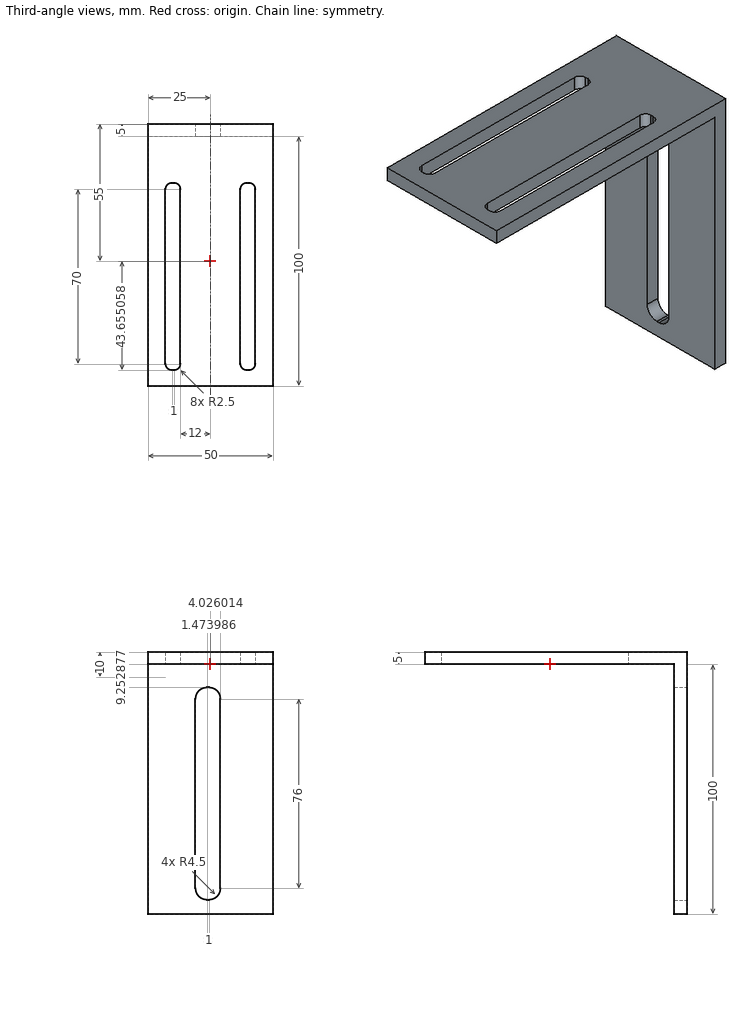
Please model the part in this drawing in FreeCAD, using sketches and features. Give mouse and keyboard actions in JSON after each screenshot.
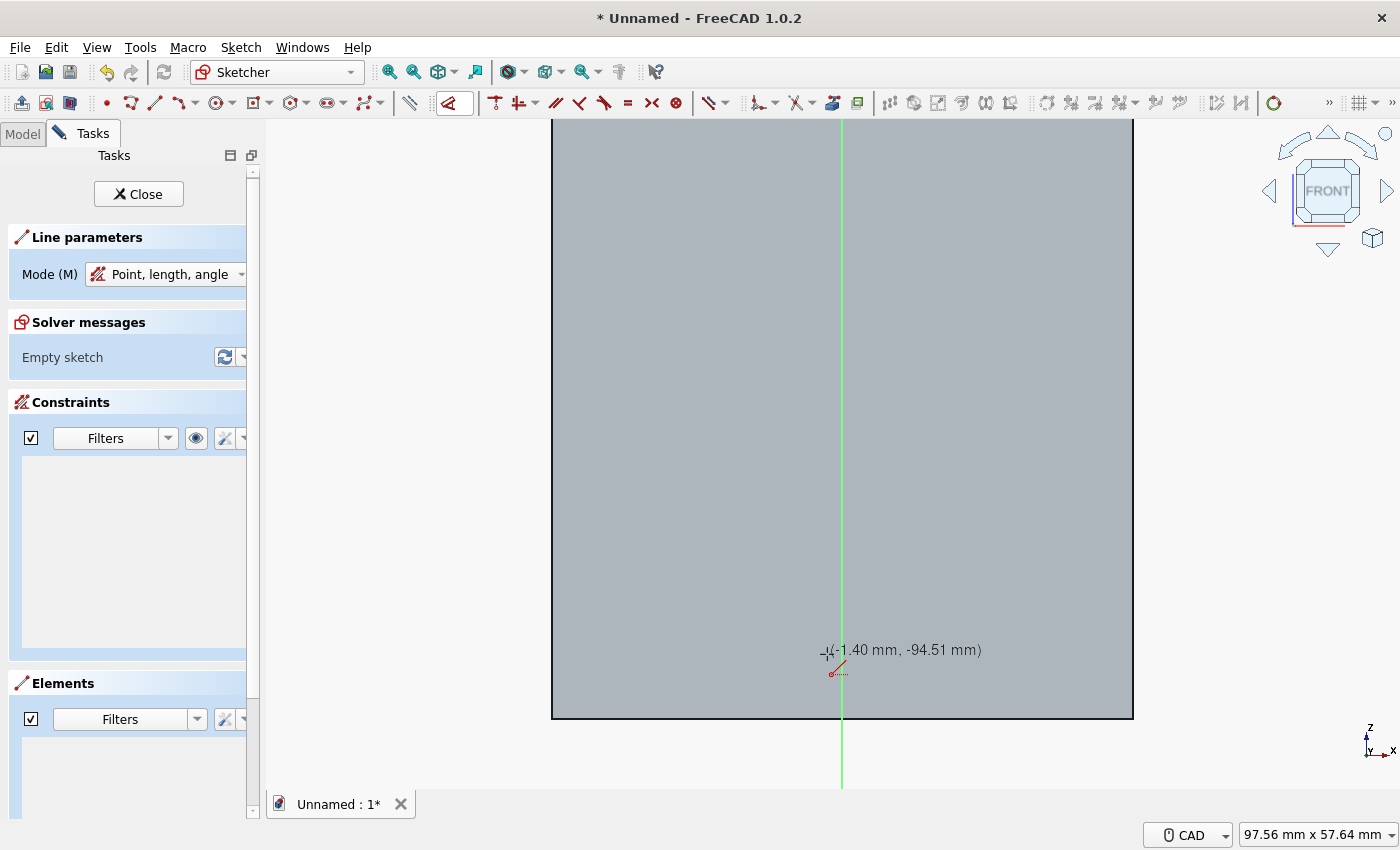
{"action": "left_click", "coordinate": [825, 652]}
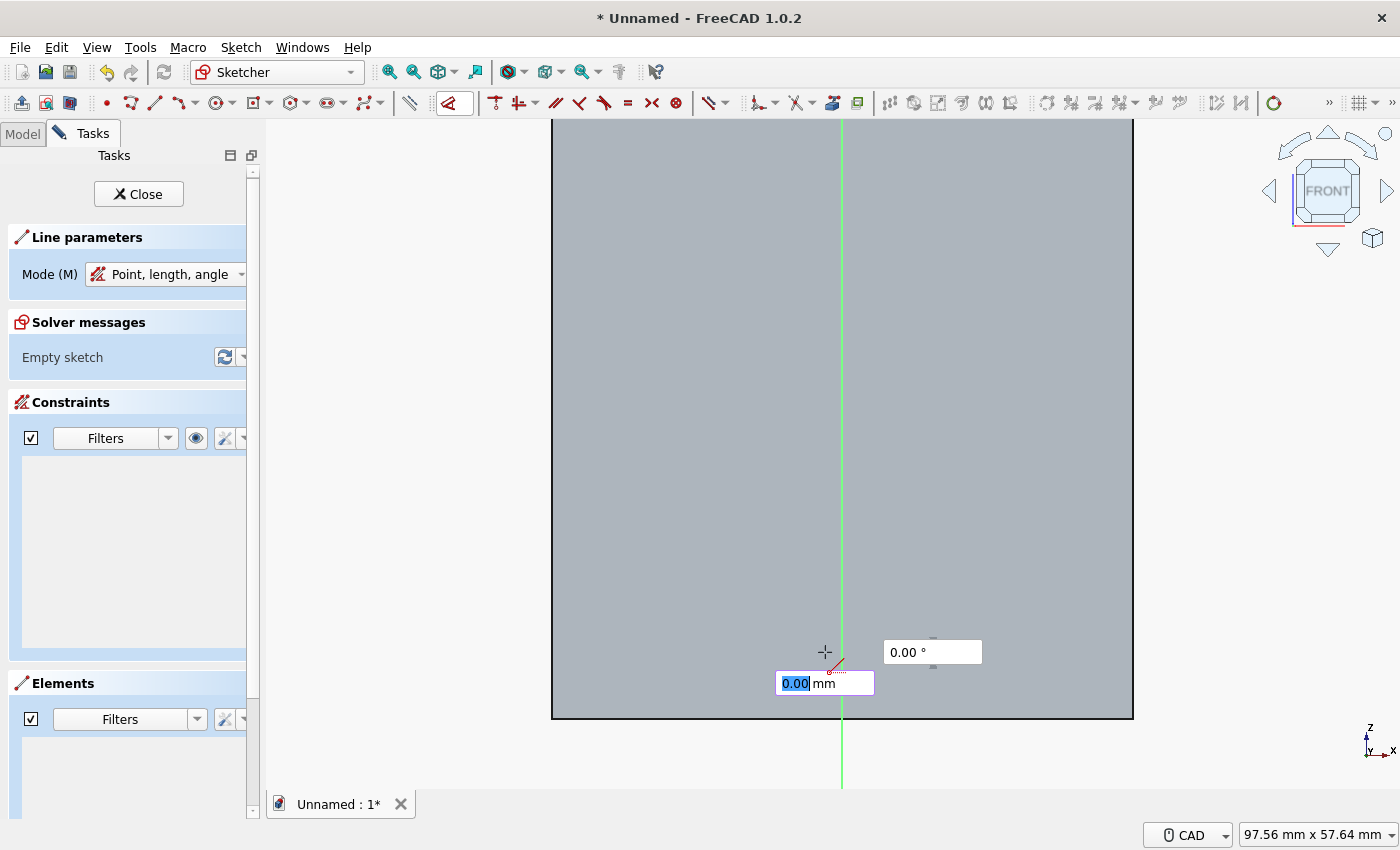
{"action": "scroll", "coordinate": [837, 652], "scroll_direction": "up", "scroll_amount": 6}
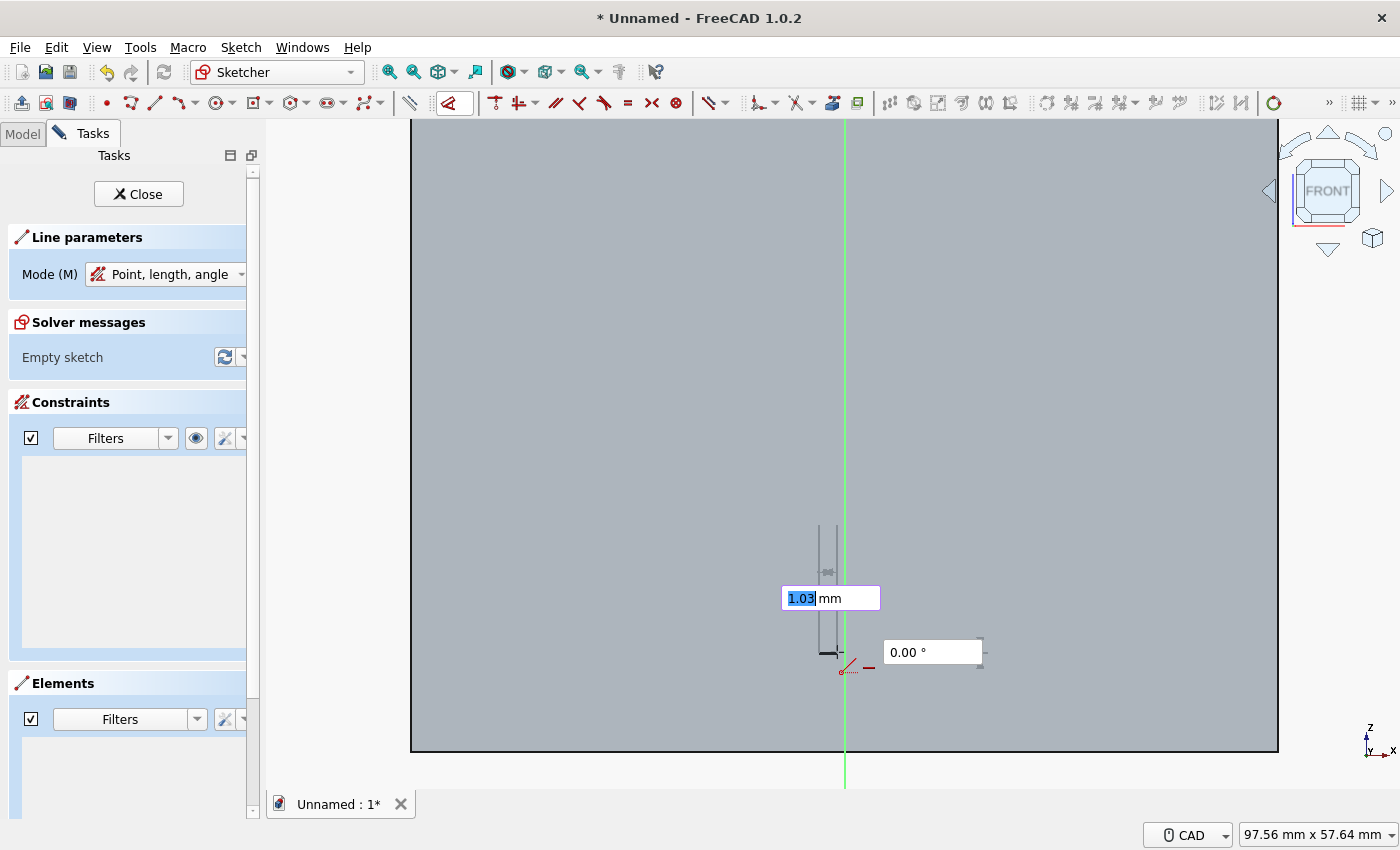
{"action": "left_click", "coordinate": [836, 650]}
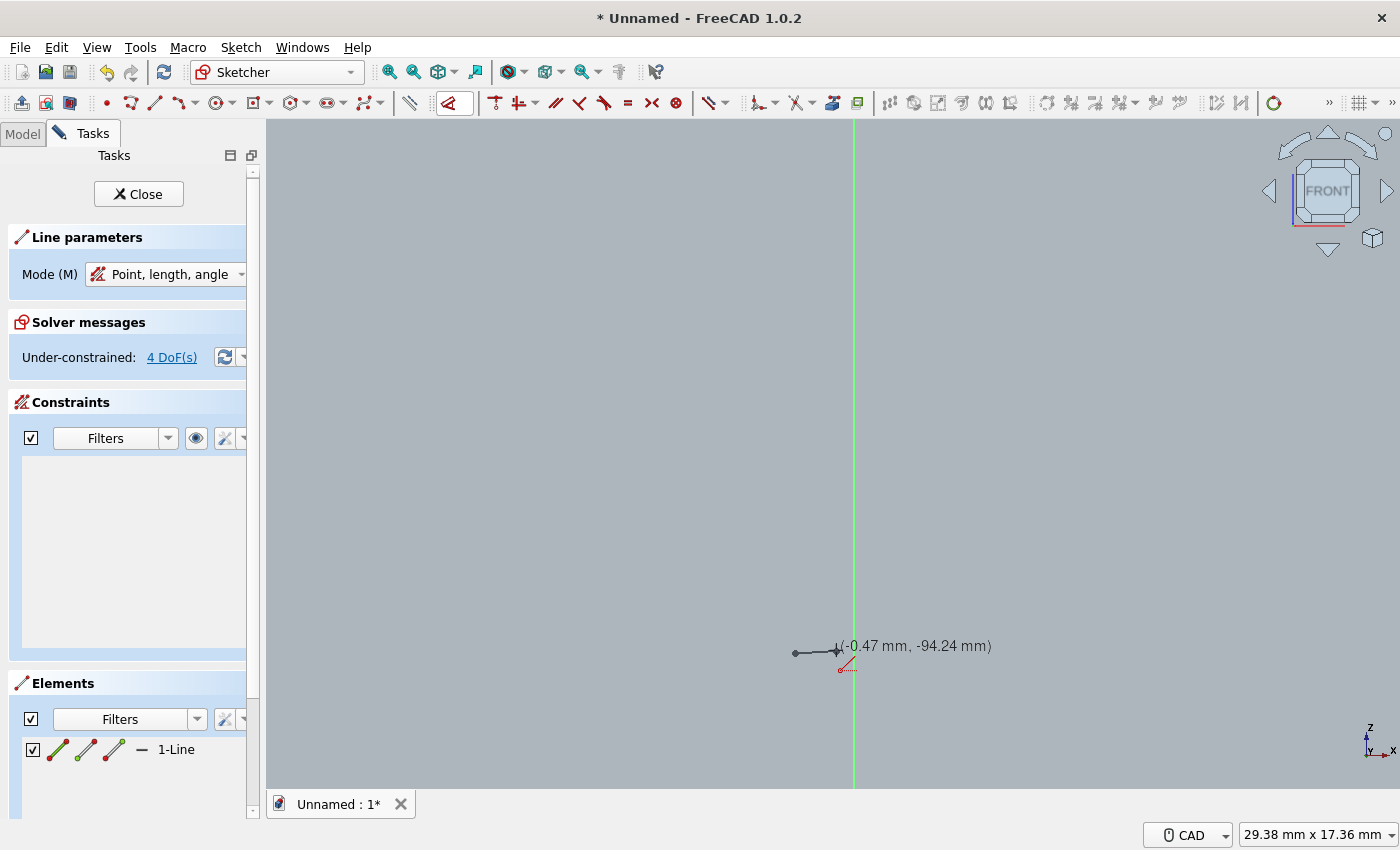
{"action": "scroll", "coordinate": [758, 656], "scroll_direction": "down", "scroll_amount": 11}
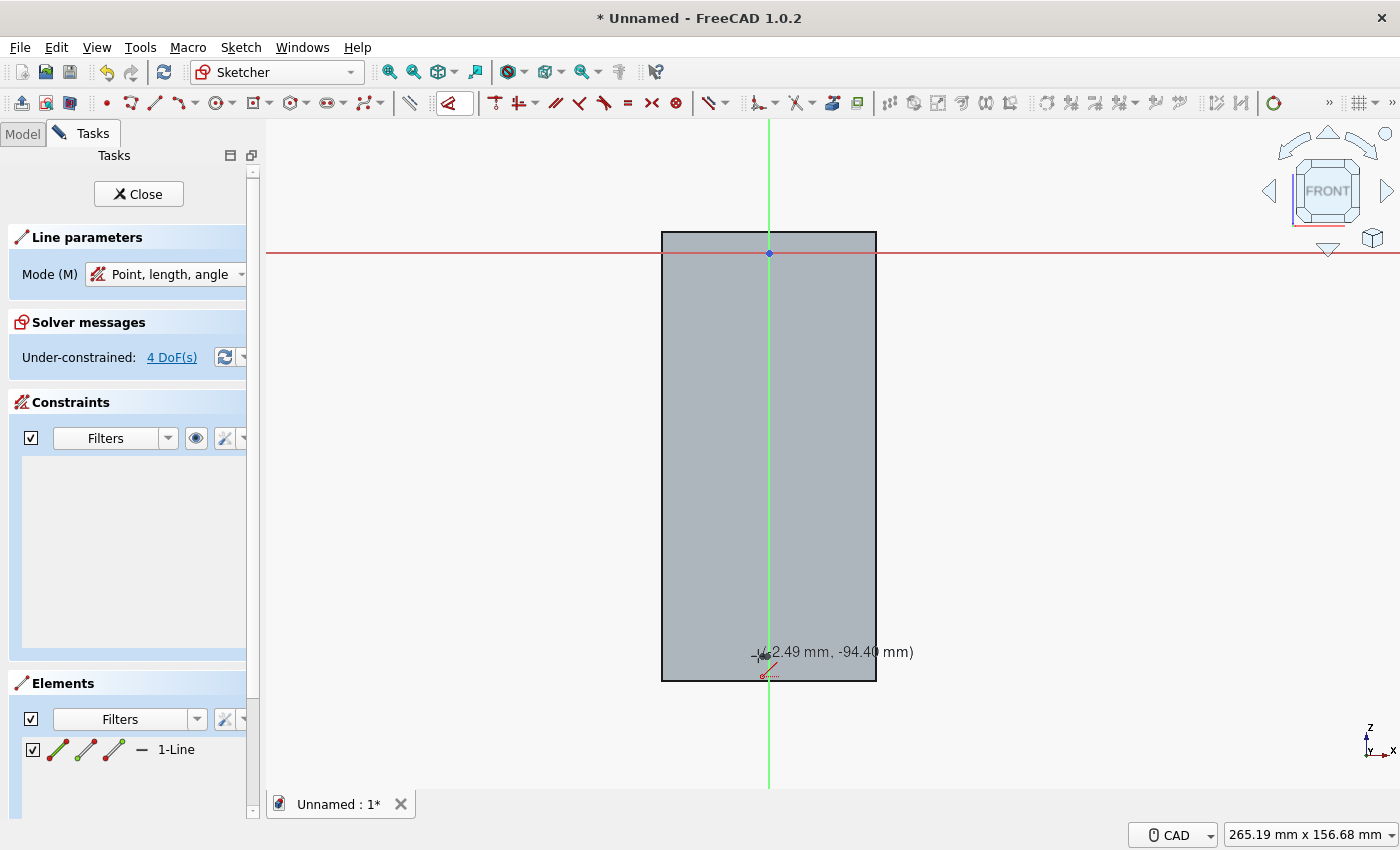
{"action": "left_click", "coordinate": [786, 637]}
{"action": "left_click", "coordinate": [786, 312]}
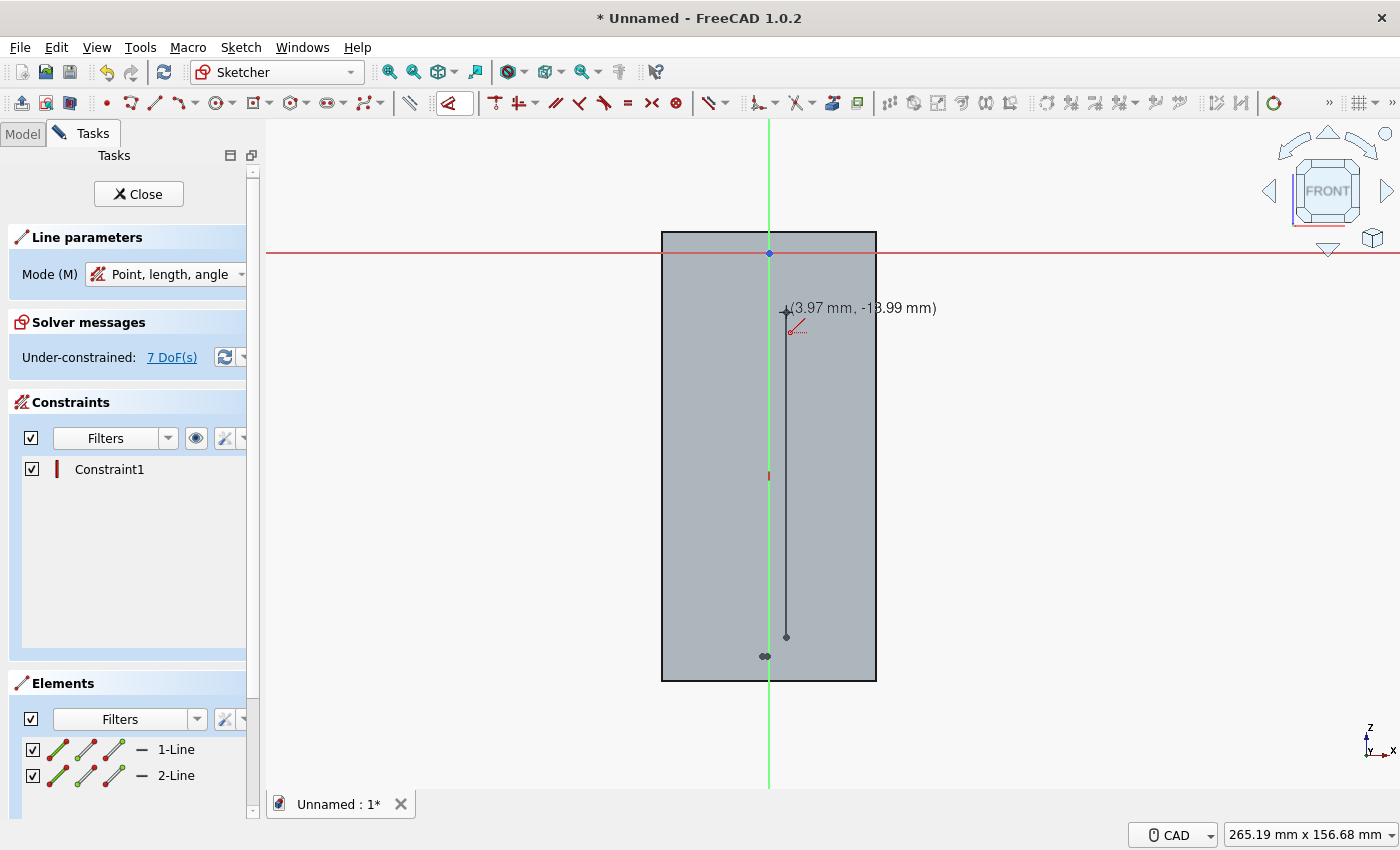
{"action": "scroll", "coordinate": [767, 293], "scroll_direction": "up", "scroll_amount": 11}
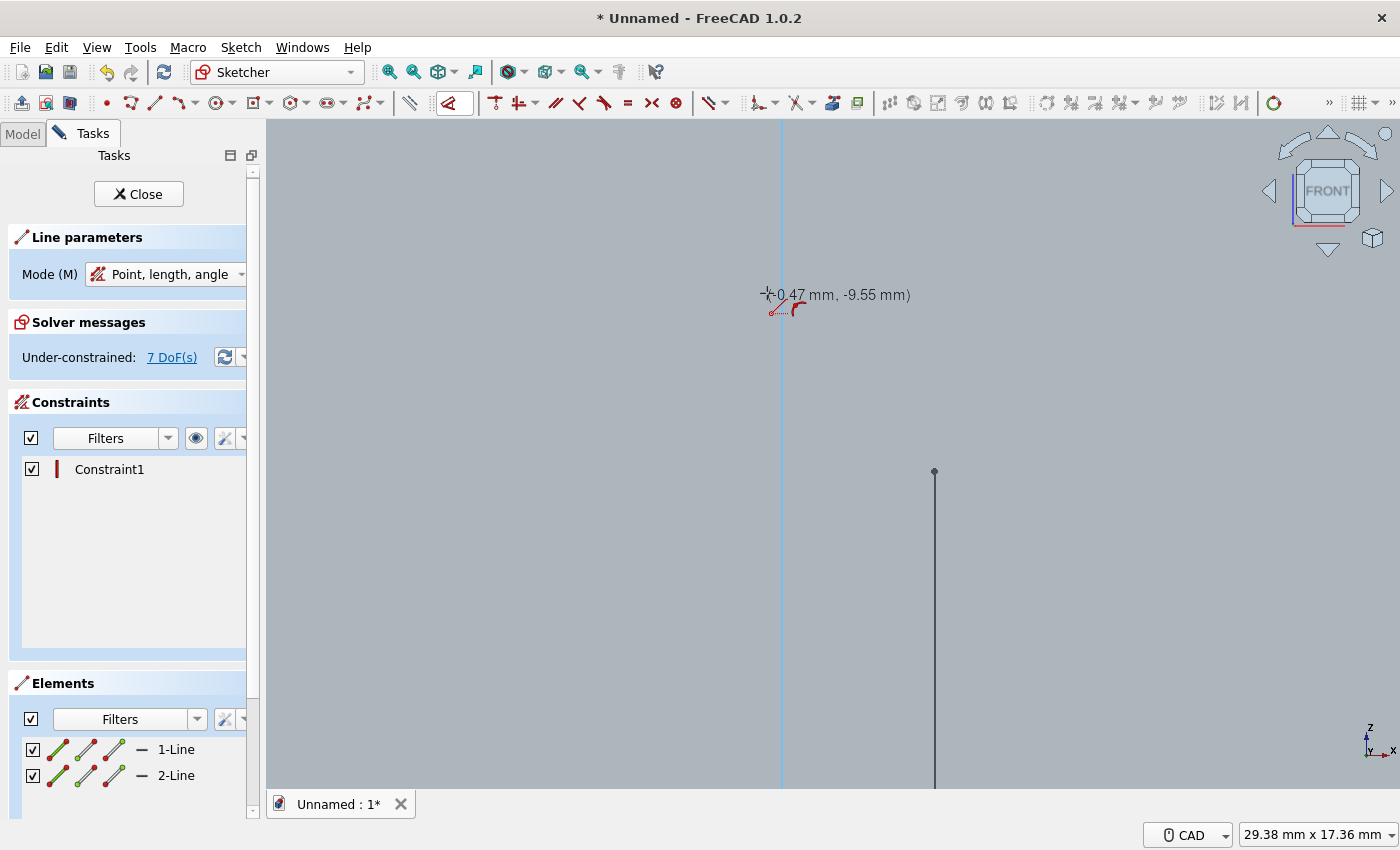
{"action": "left_click", "coordinate": [763, 289]}
{"action": "left_click", "coordinate": [725, 289]}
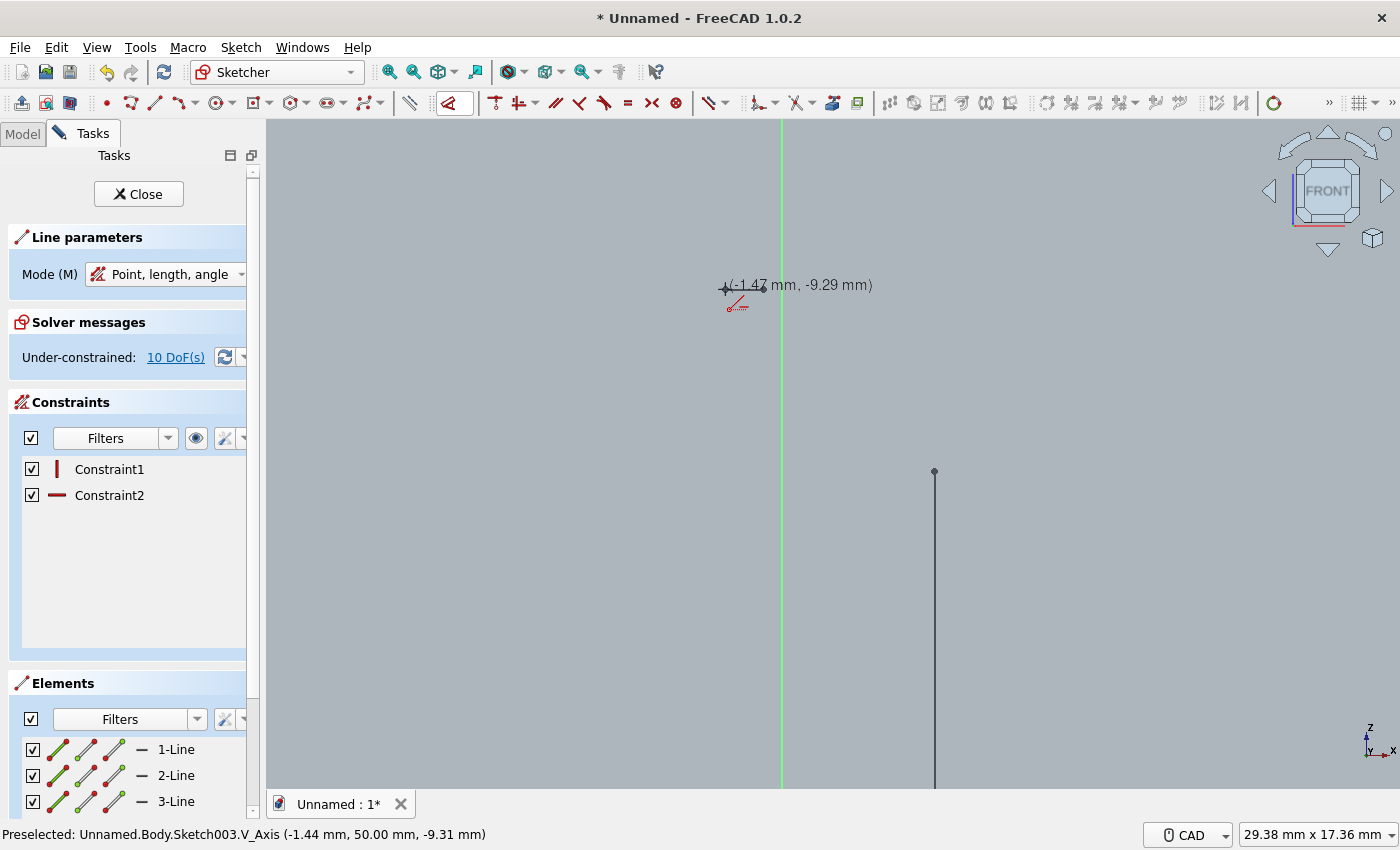
{"action": "scroll", "coordinate": [767, 292], "scroll_direction": "down", "scroll_amount": 11}